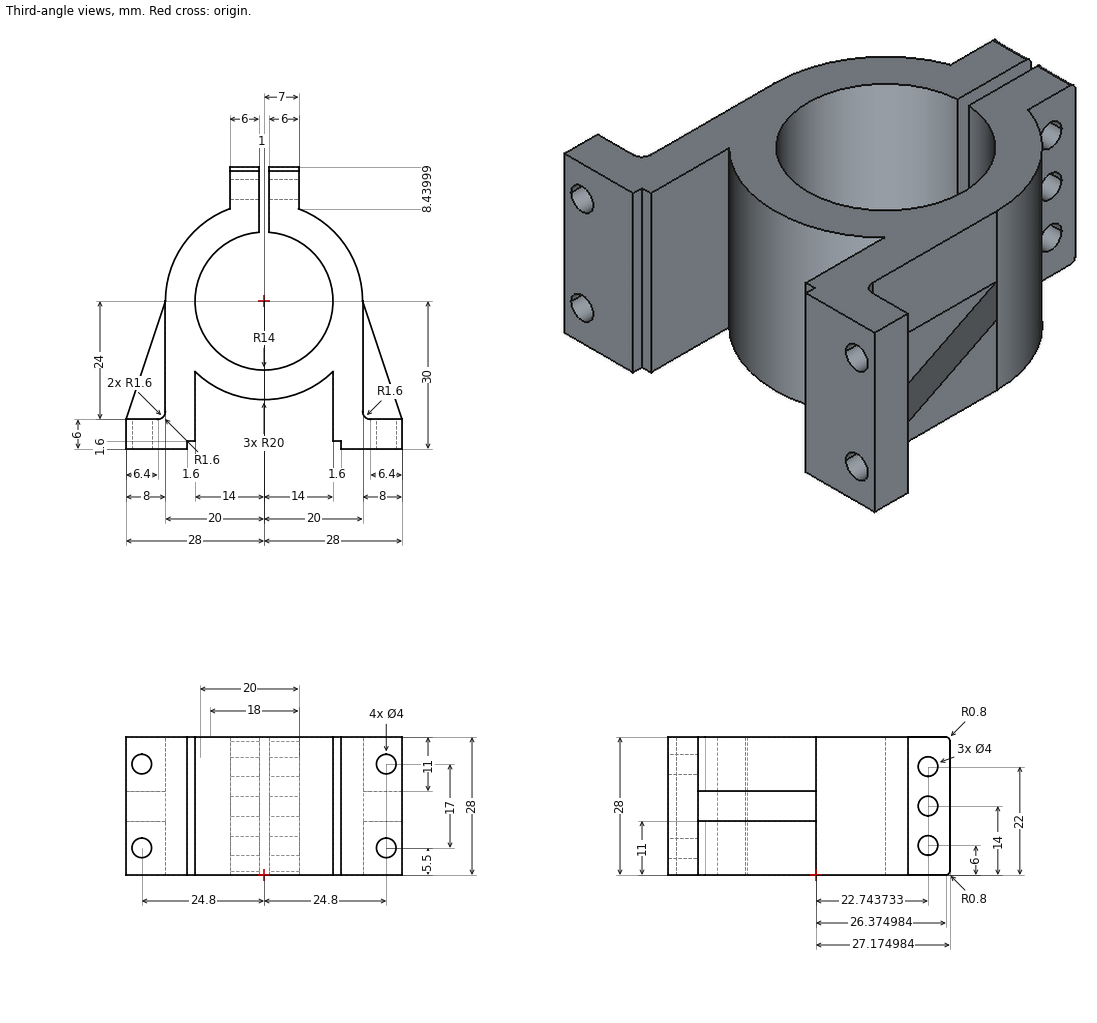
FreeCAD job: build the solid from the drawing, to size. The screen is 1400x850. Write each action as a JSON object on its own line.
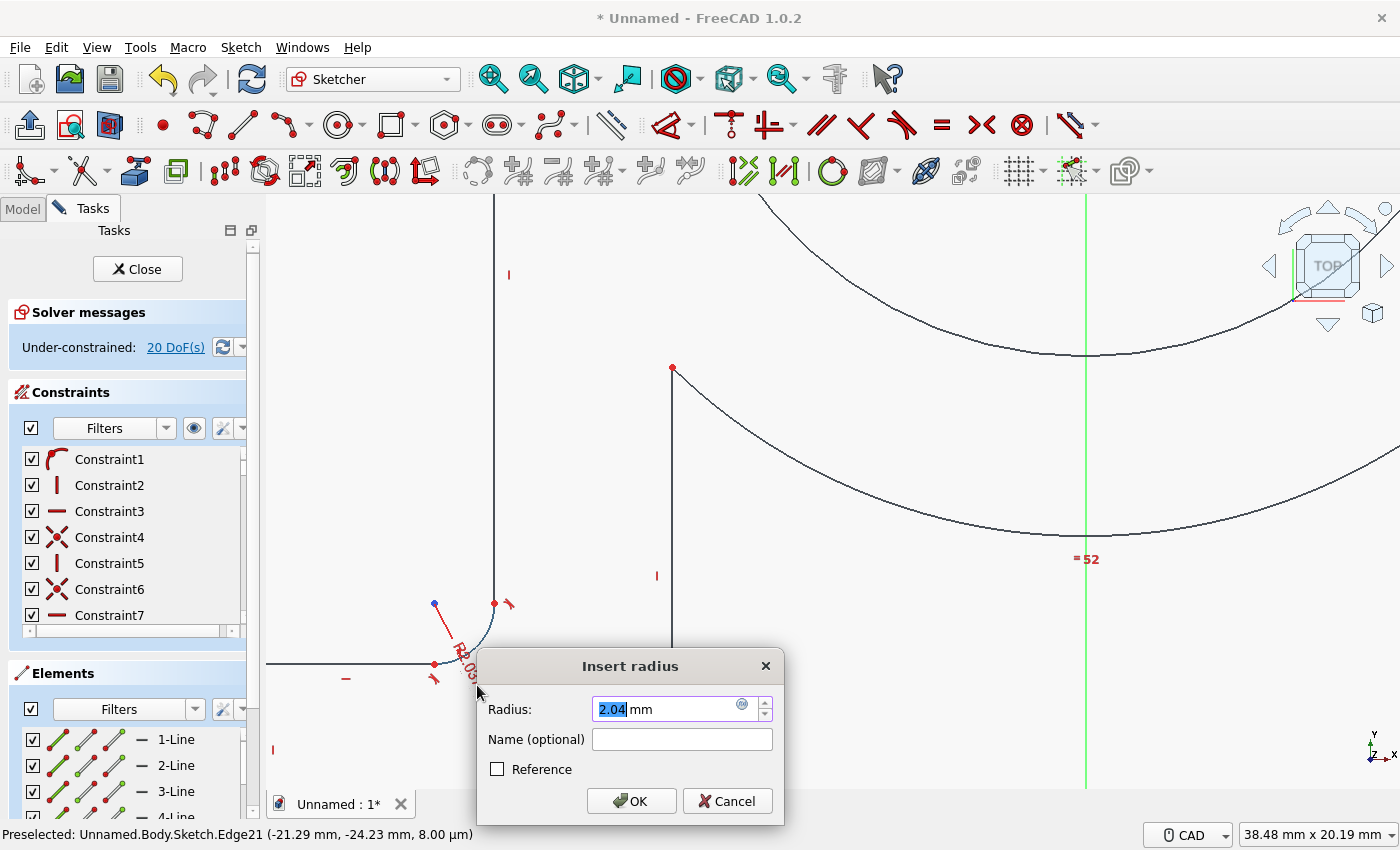
{"action": "type", "text": "1.6"}
{"action": "key", "text": "Return"}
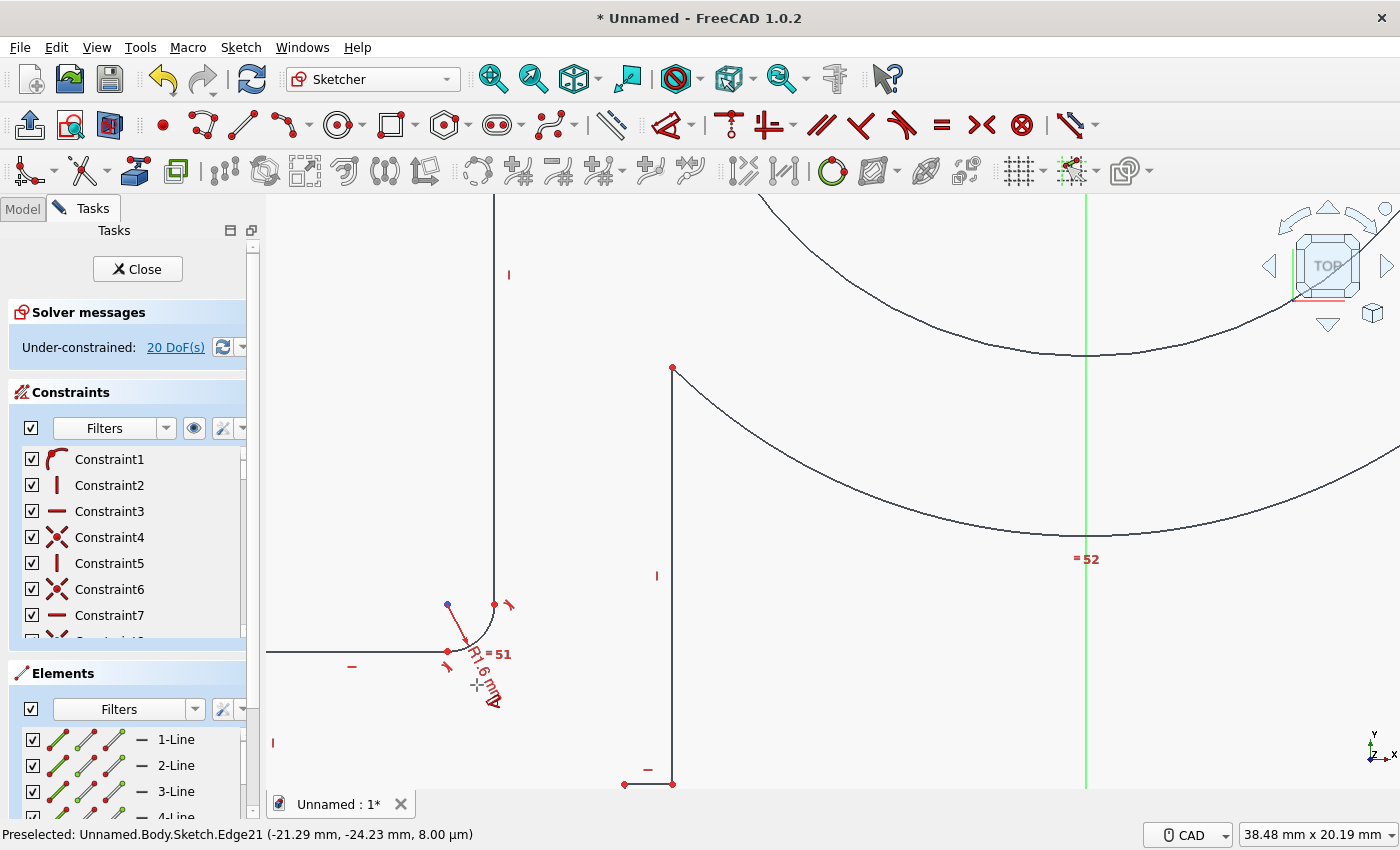
{"action": "scroll", "coordinate": [659, 657], "scroll_direction": "down", "scroll_amount": 7}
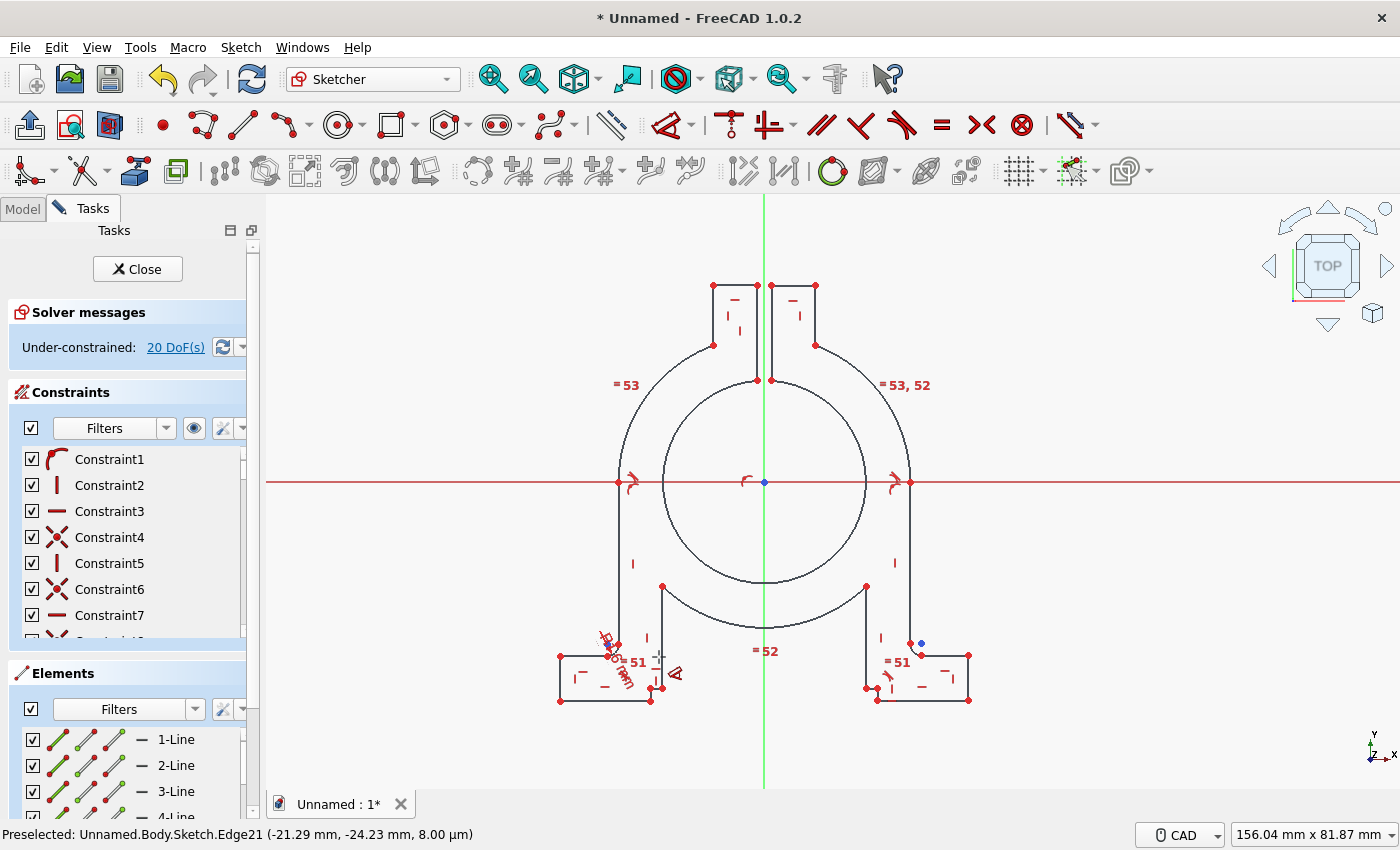
{"action": "left_click", "coordinate": [720, 621]}
{"action": "left_click", "coordinate": [710, 651]}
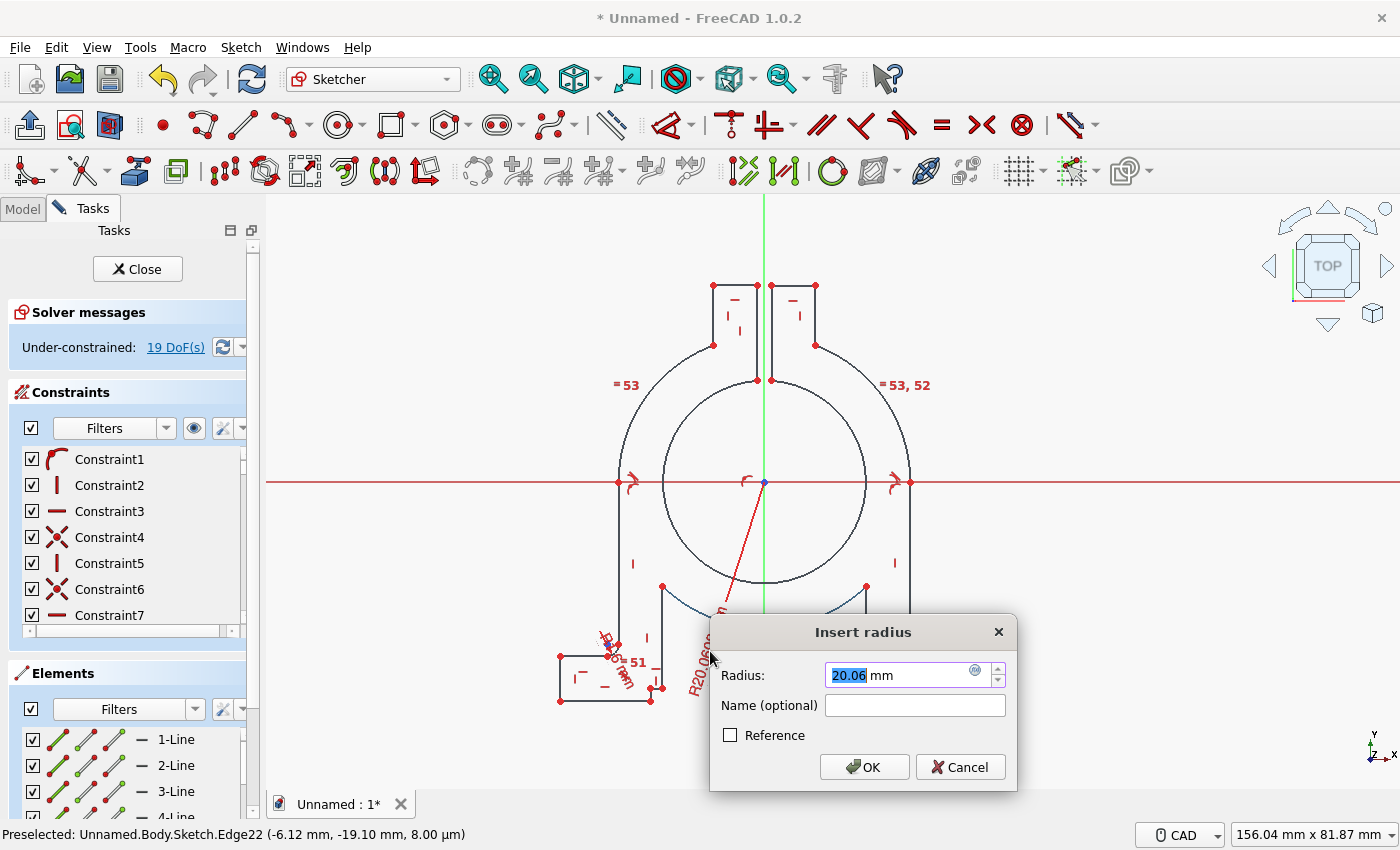
{"action": "type", "text": "20"}
{"action": "key", "text": "Return"}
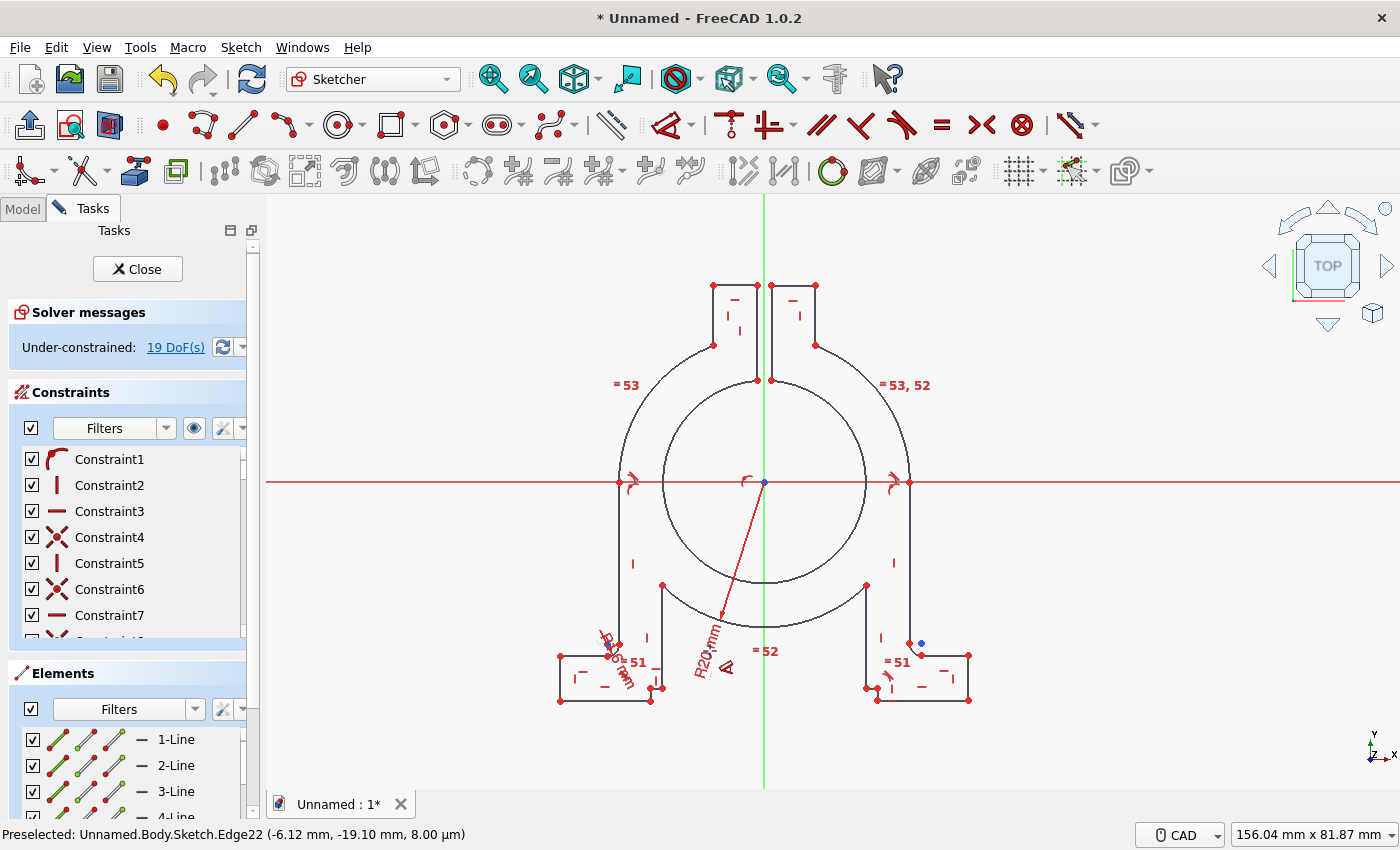
{"action": "left_click", "coordinate": [669, 516]}
{"action": "left_click", "coordinate": [639, 527]}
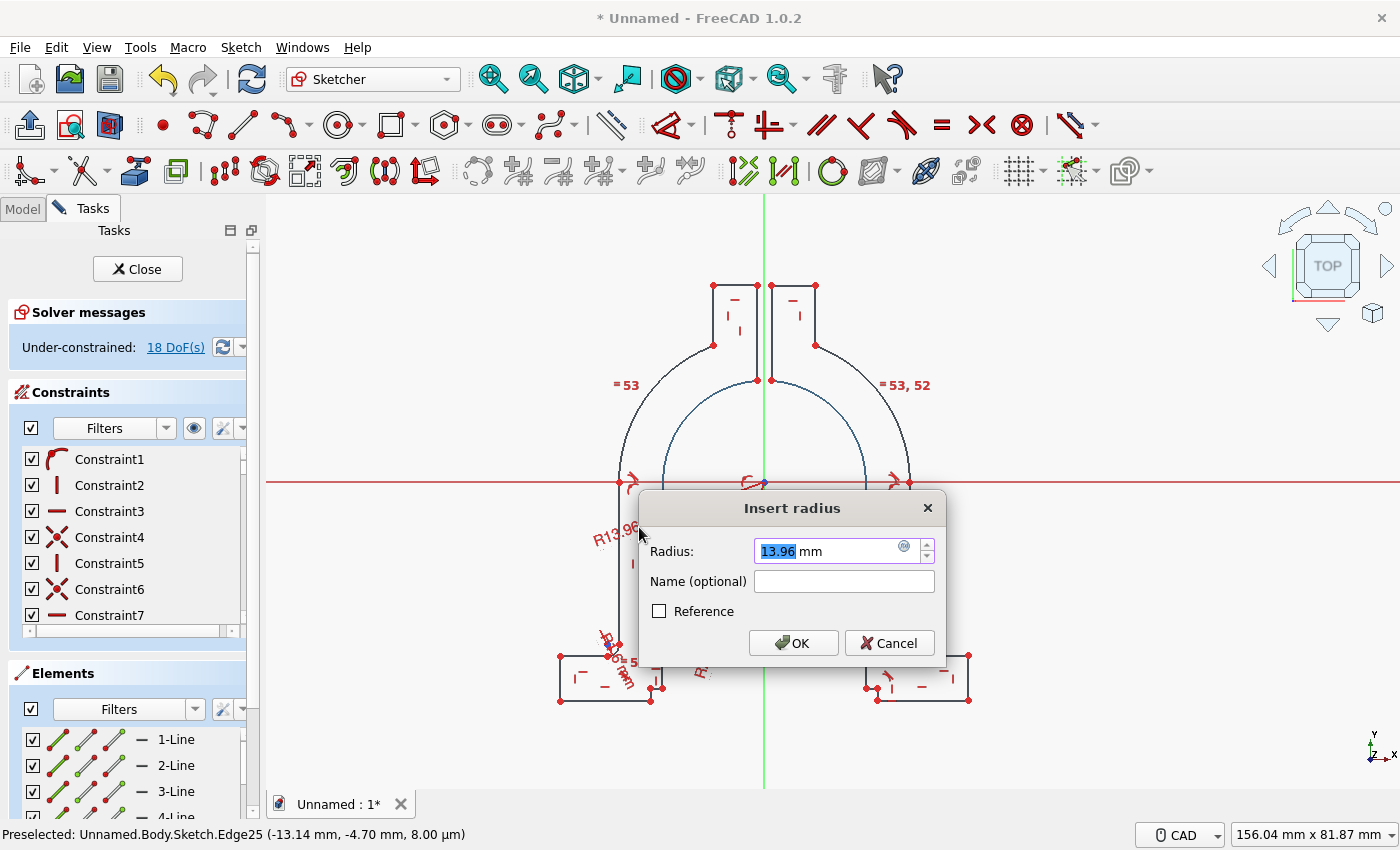
{"action": "type", "text": "14"}
{"action": "key", "text": "Return"}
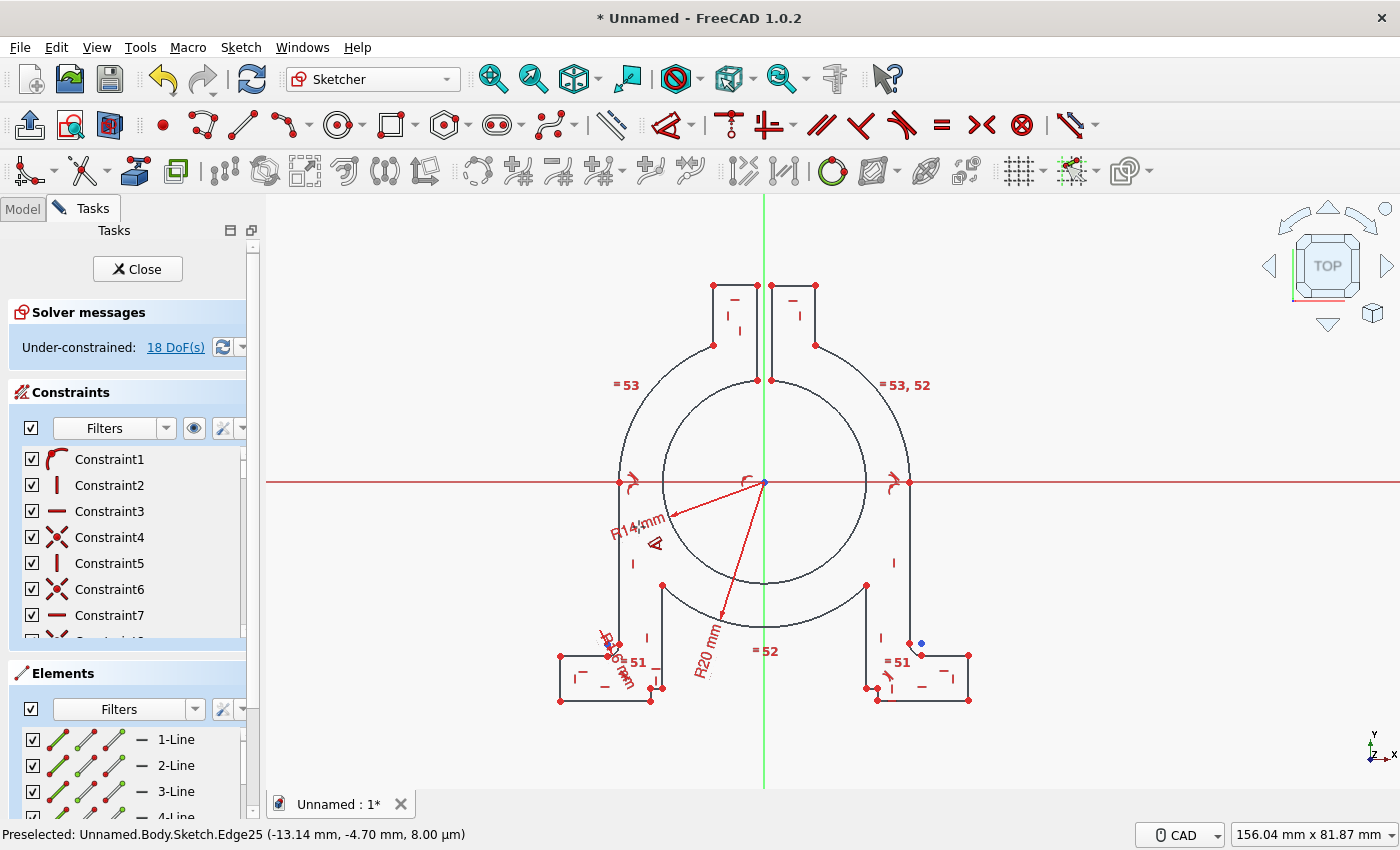
{"action": "left_click", "coordinate": [560, 670]}
{"action": "left_click", "coordinate": [526, 679]}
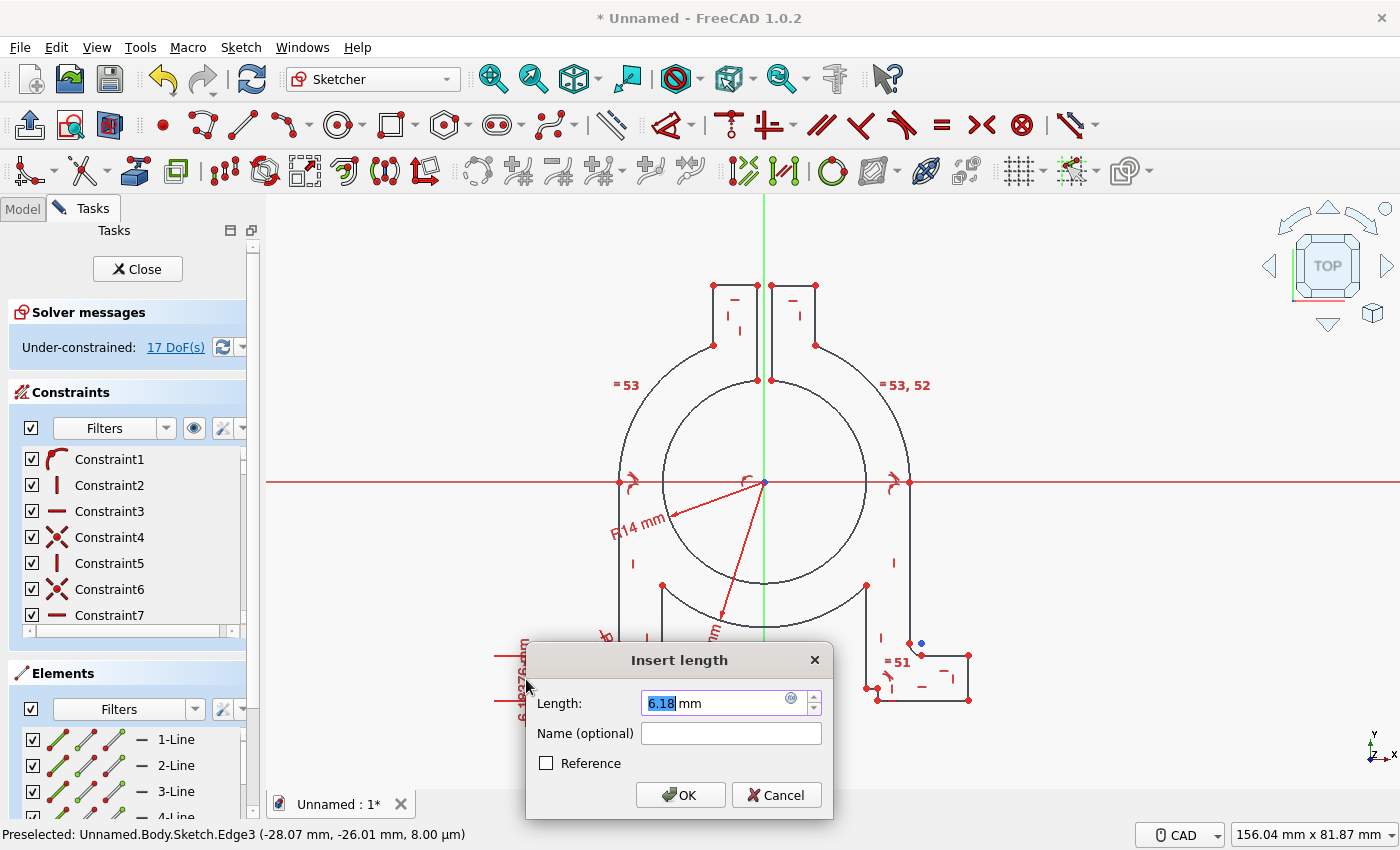
{"action": "type", "text": "6"}
{"action": "key", "text": "Return"}